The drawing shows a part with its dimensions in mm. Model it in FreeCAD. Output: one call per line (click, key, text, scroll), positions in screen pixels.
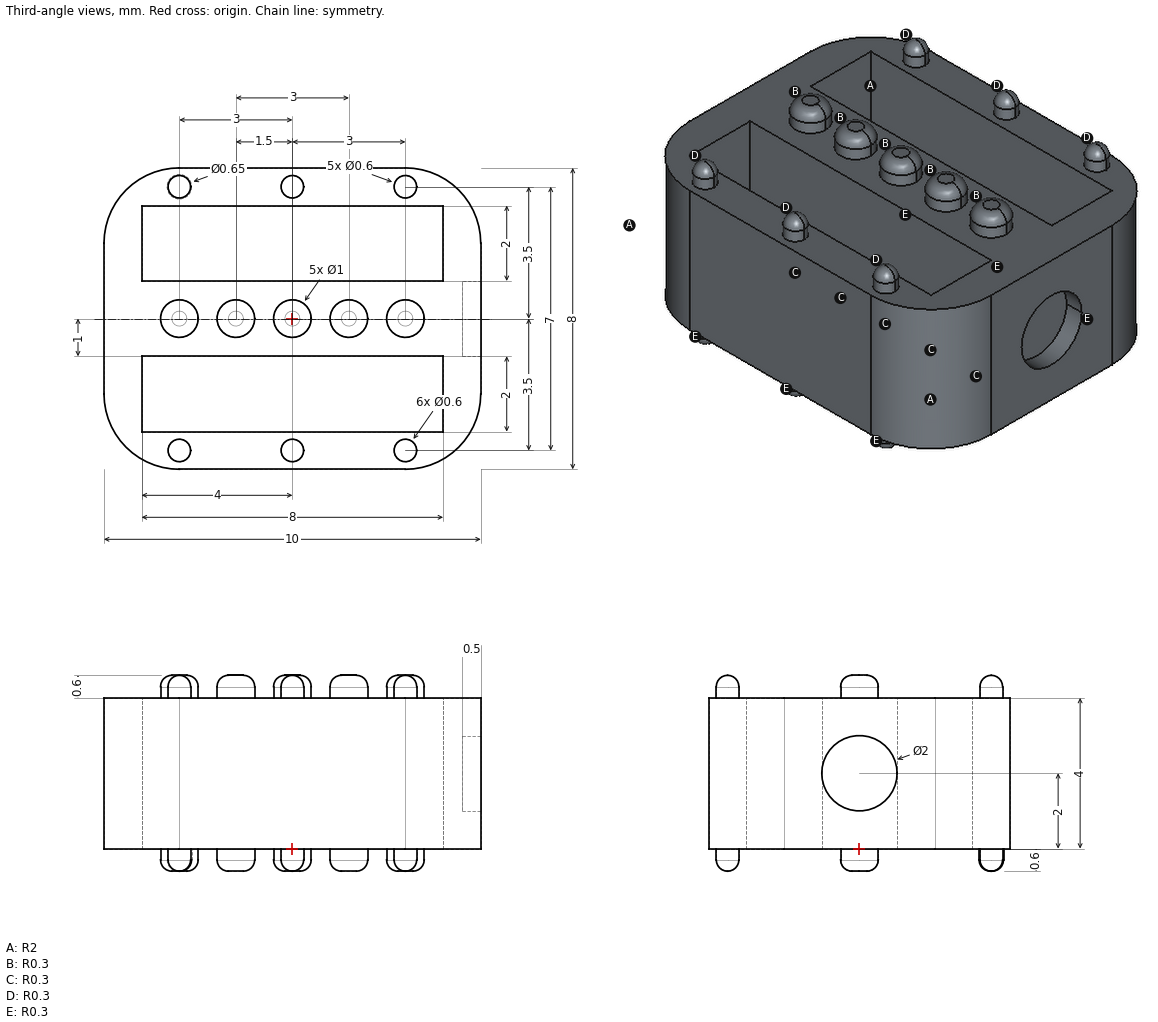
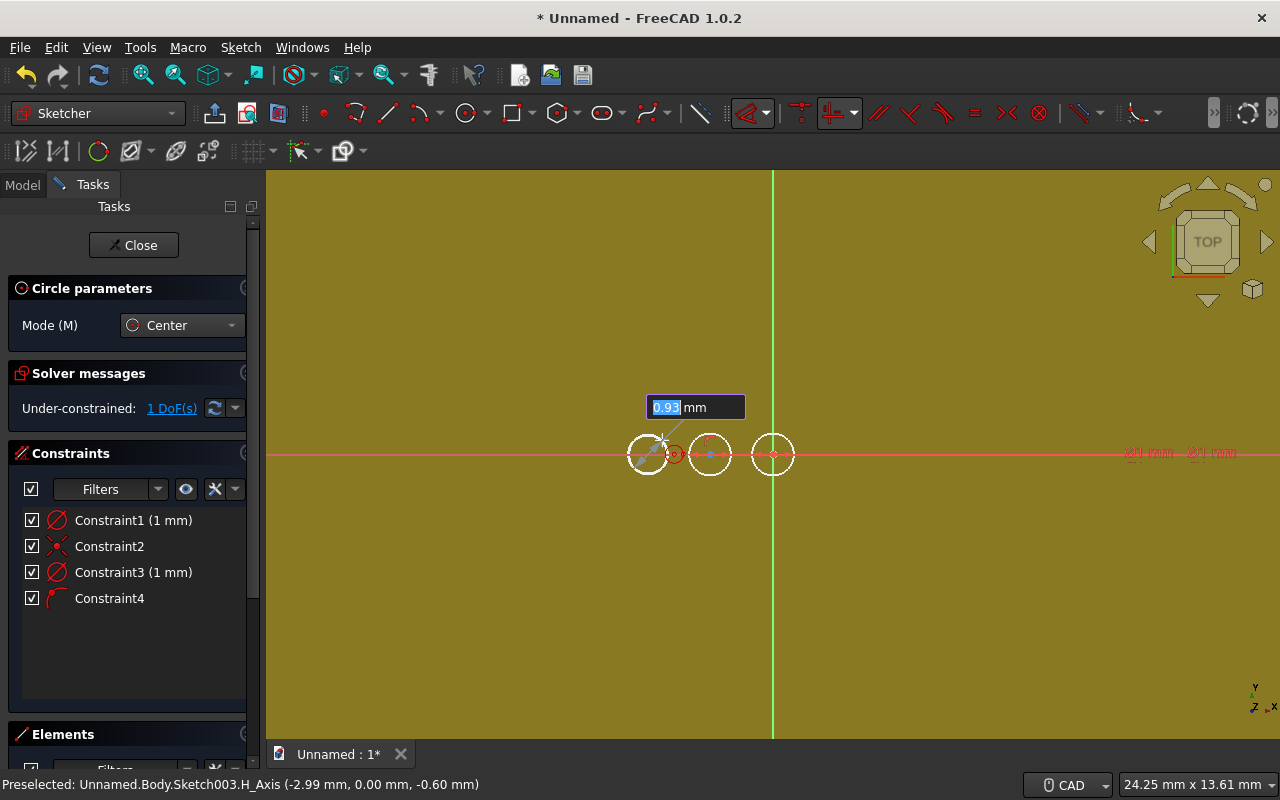
text(1)
key(Return)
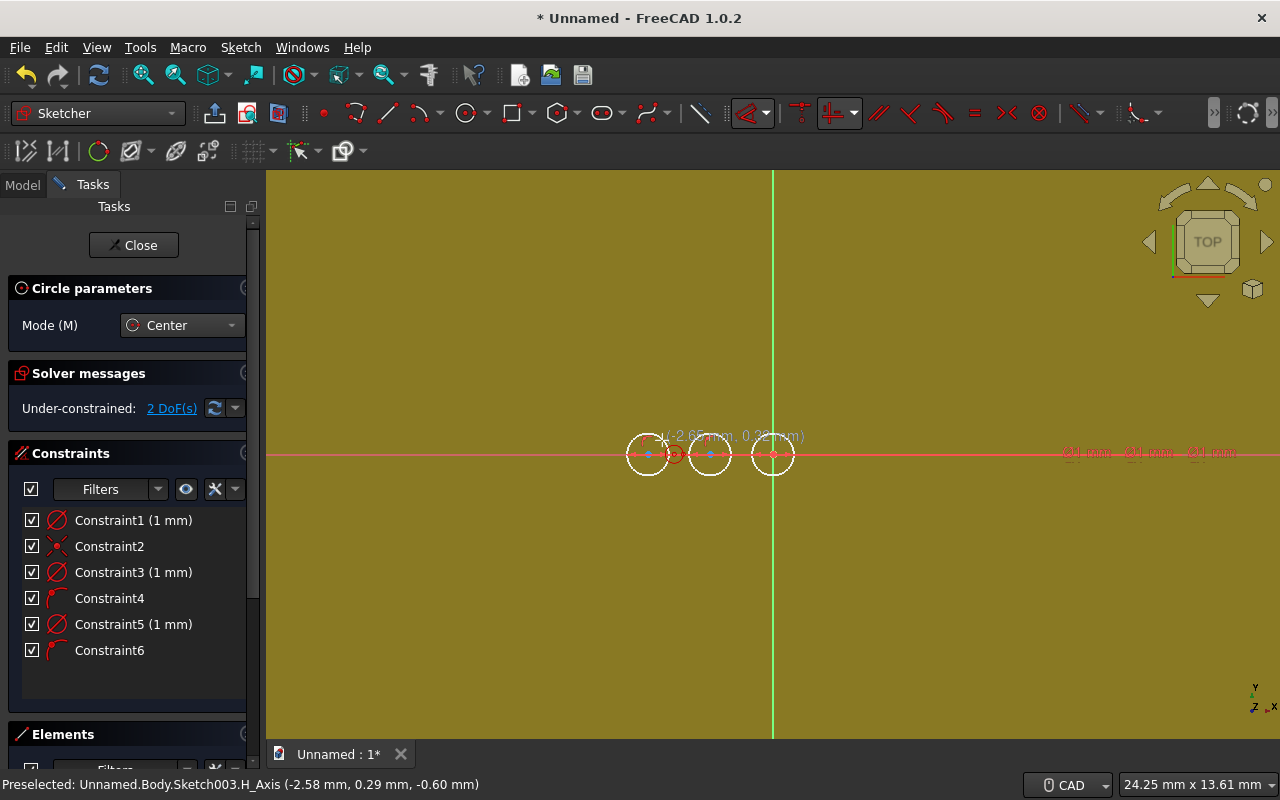
click(836, 454)
move(851, 440)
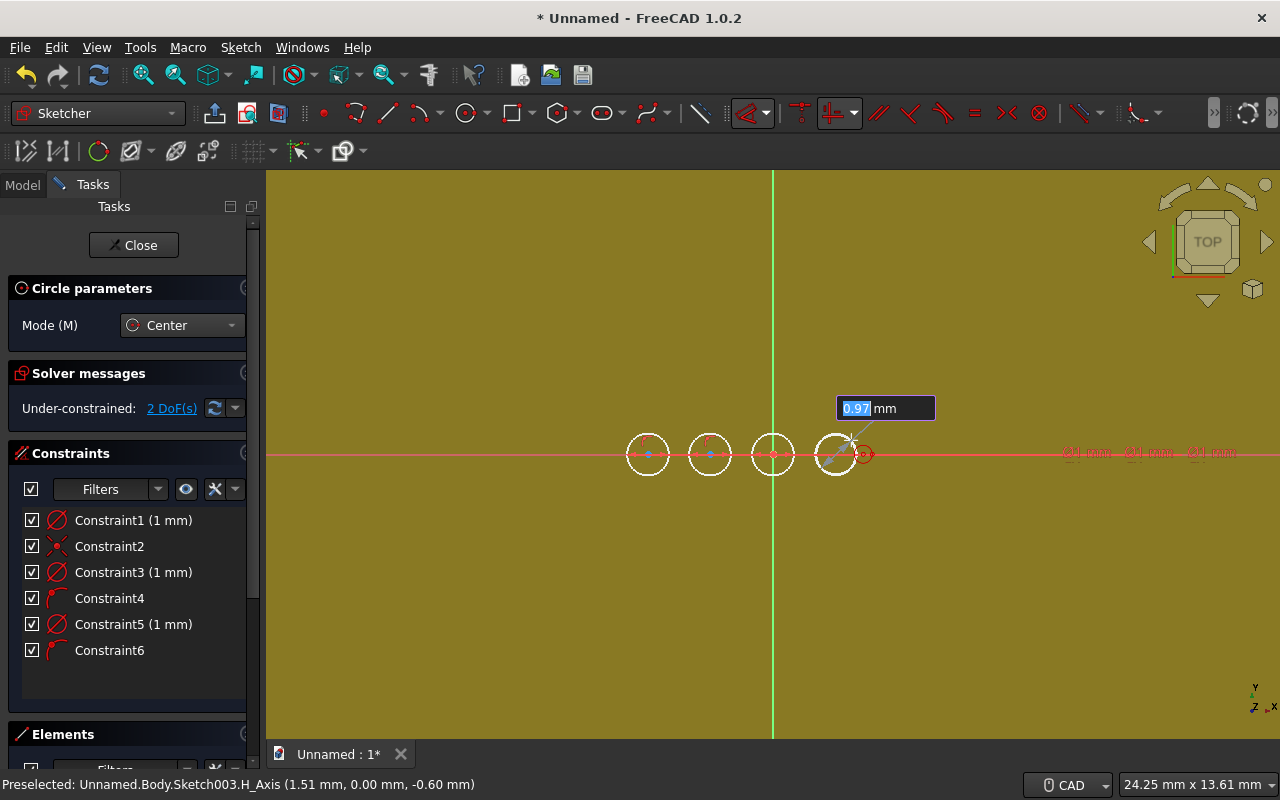
text(1)
key(Return)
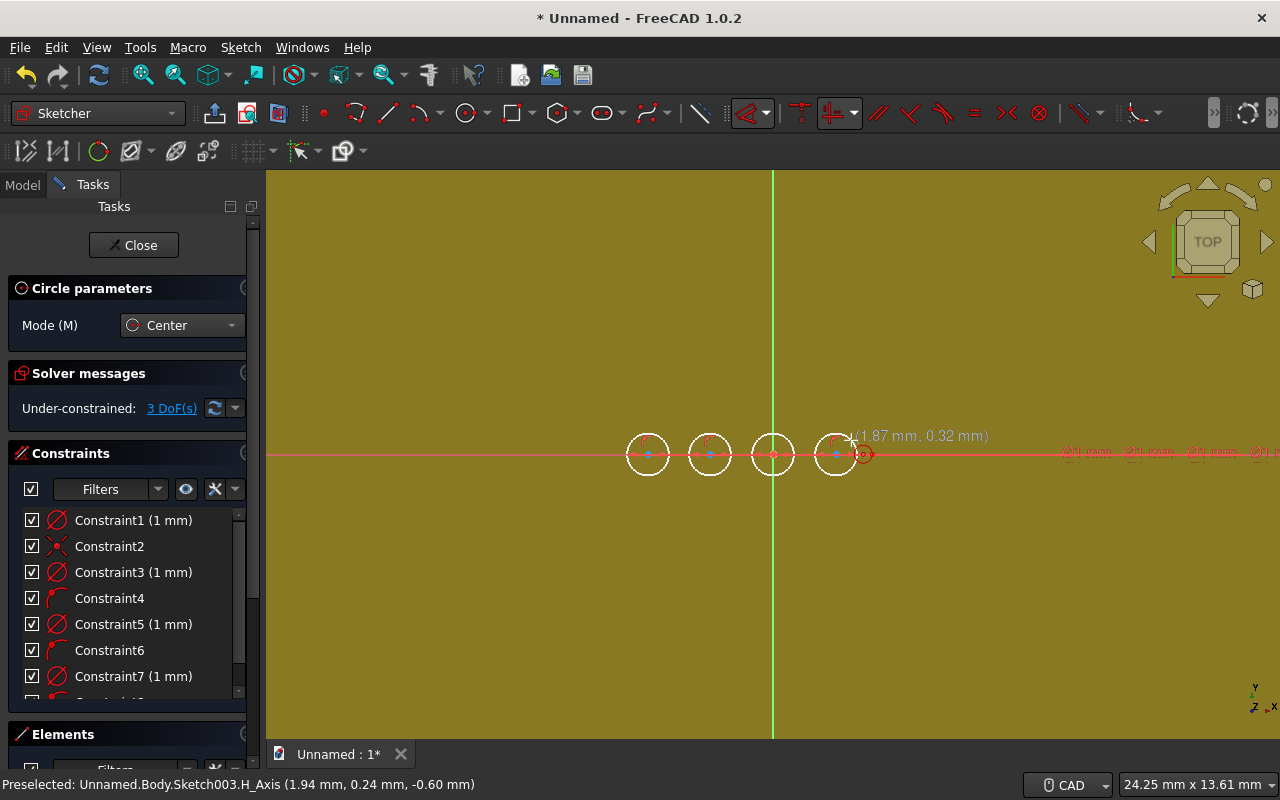
click(898, 454)
move(913, 440)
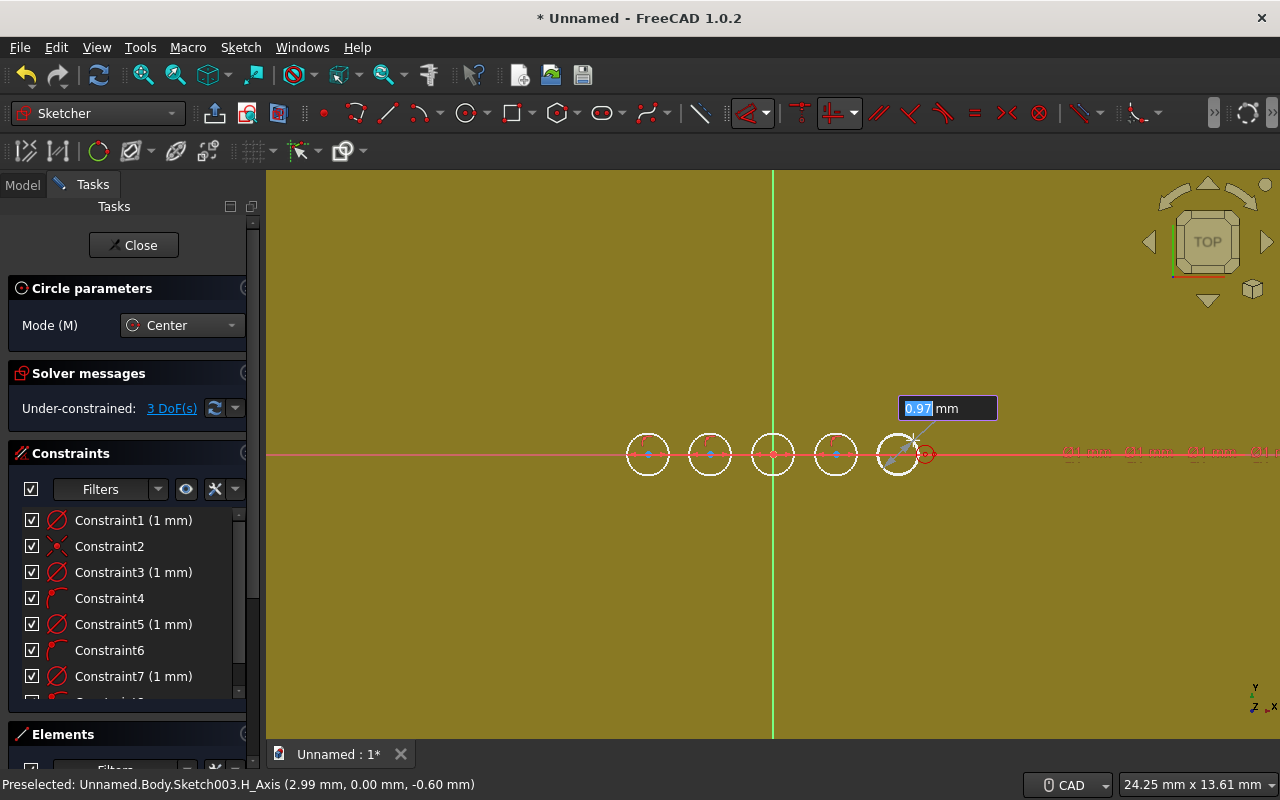
text(1)
key(Return)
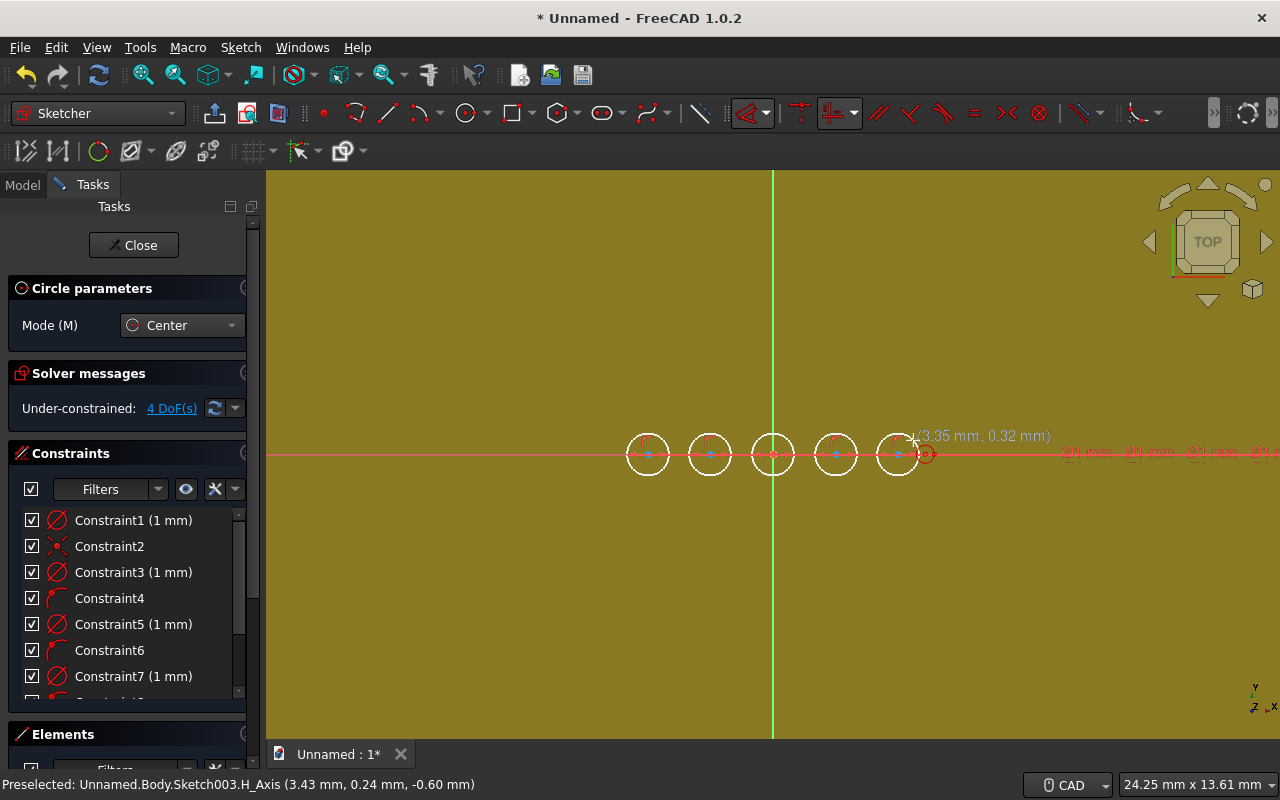
scroll(898, 308, up, 3)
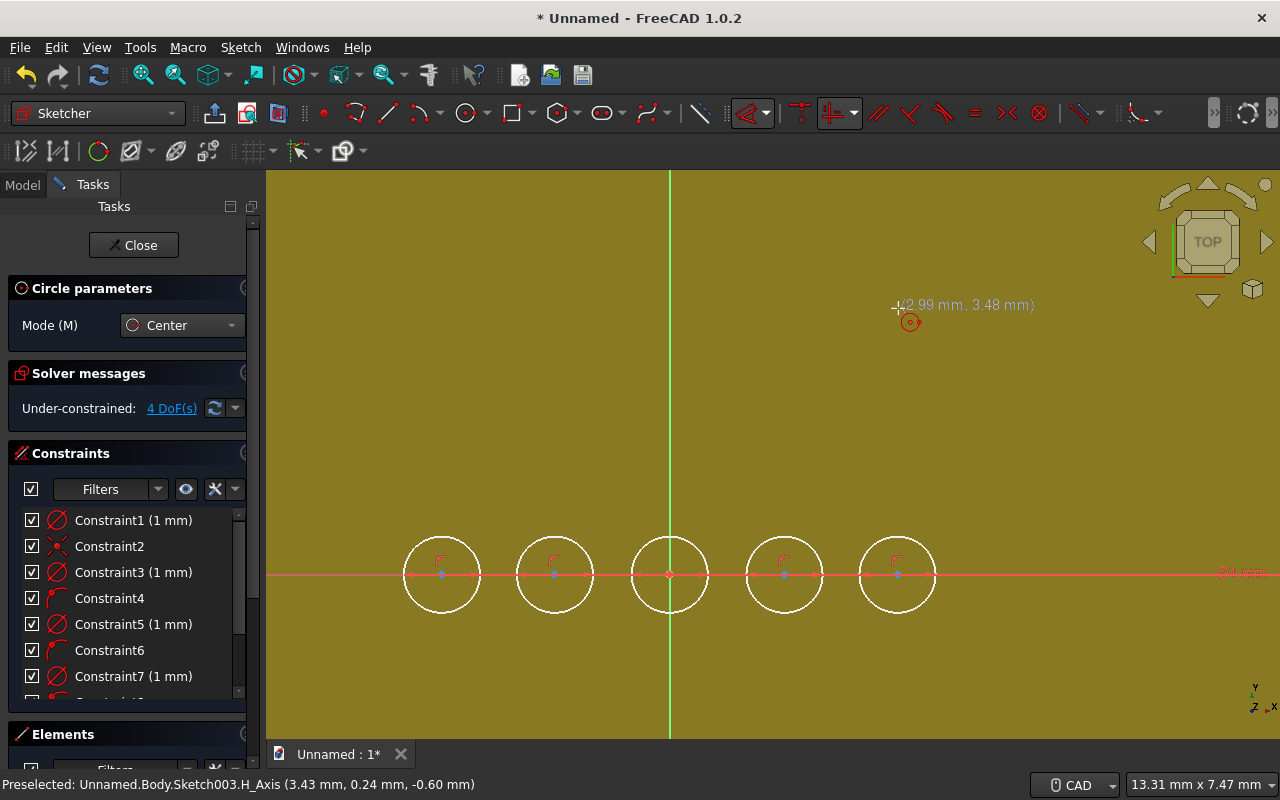
click(898, 308)
move(914, 292)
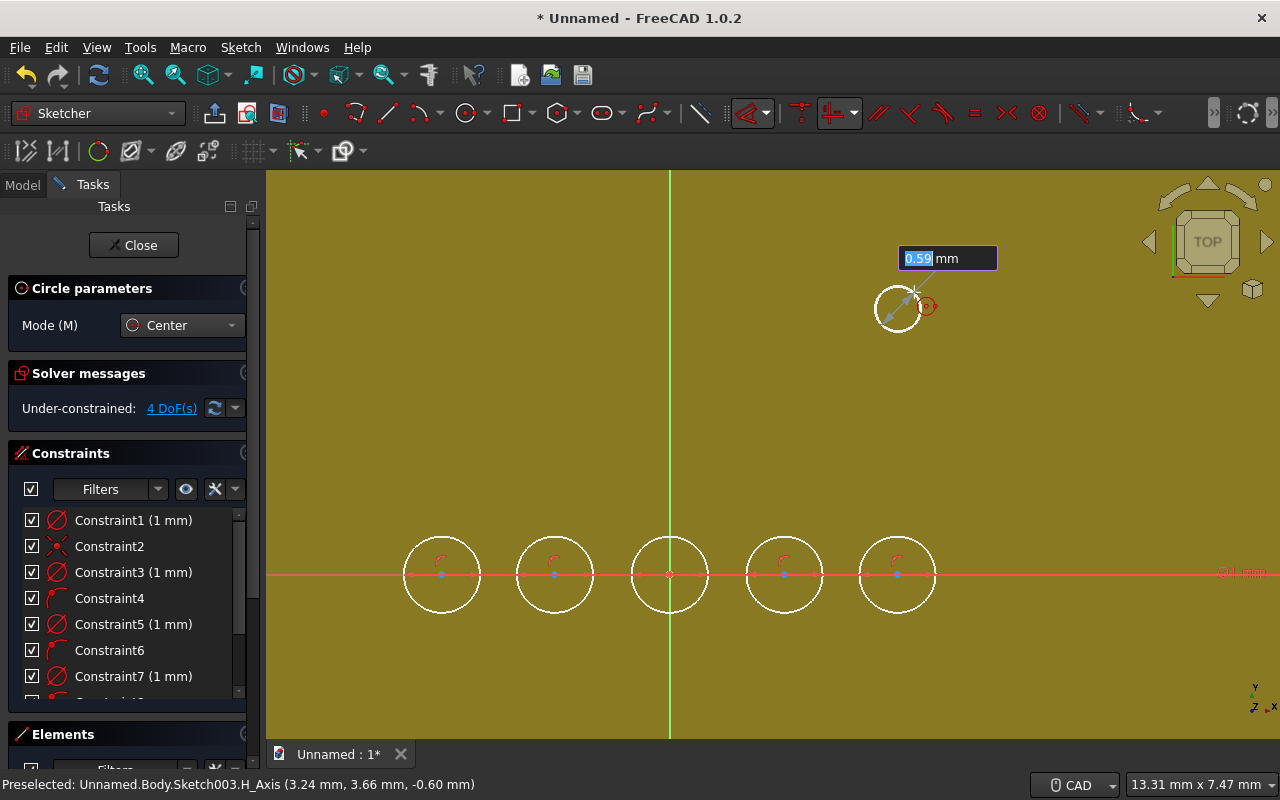
text(0.6)
key(Return)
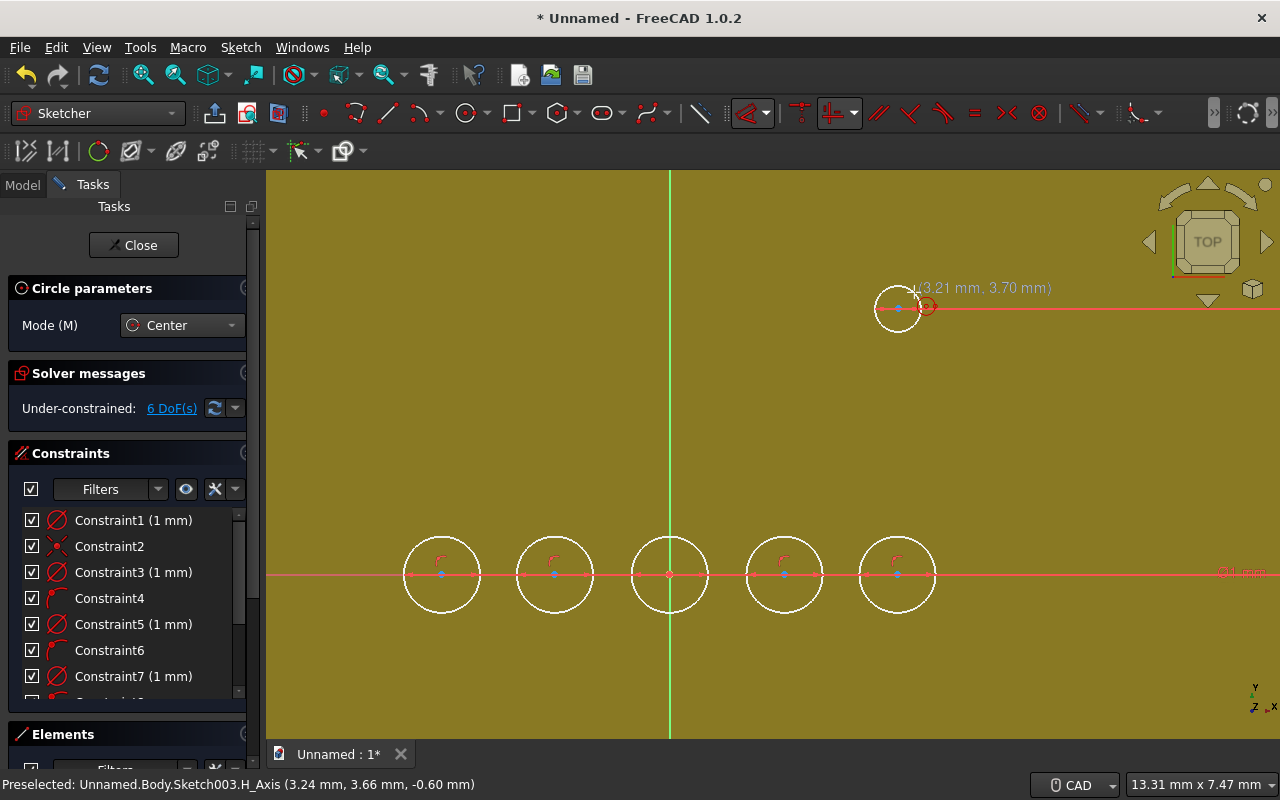
click(670, 308)
move(686, 292)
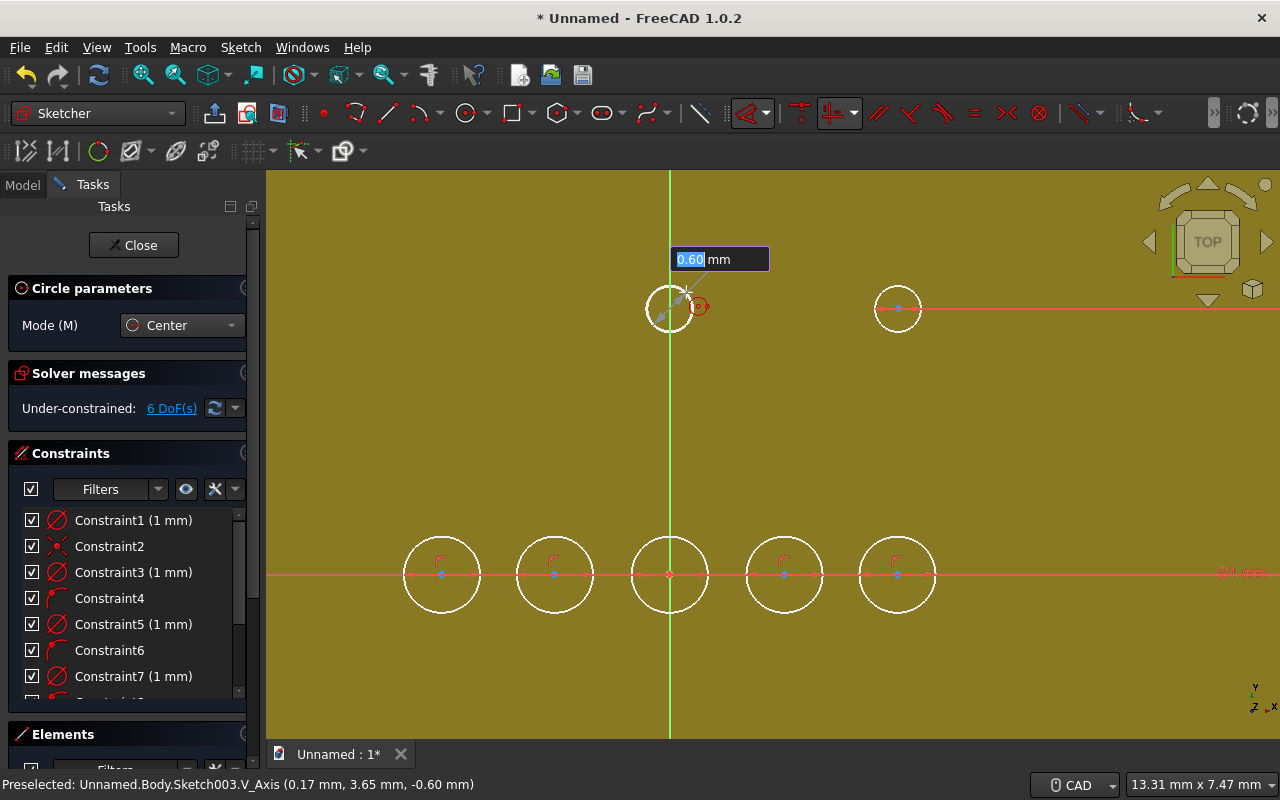
text(0.6)
key(Return)